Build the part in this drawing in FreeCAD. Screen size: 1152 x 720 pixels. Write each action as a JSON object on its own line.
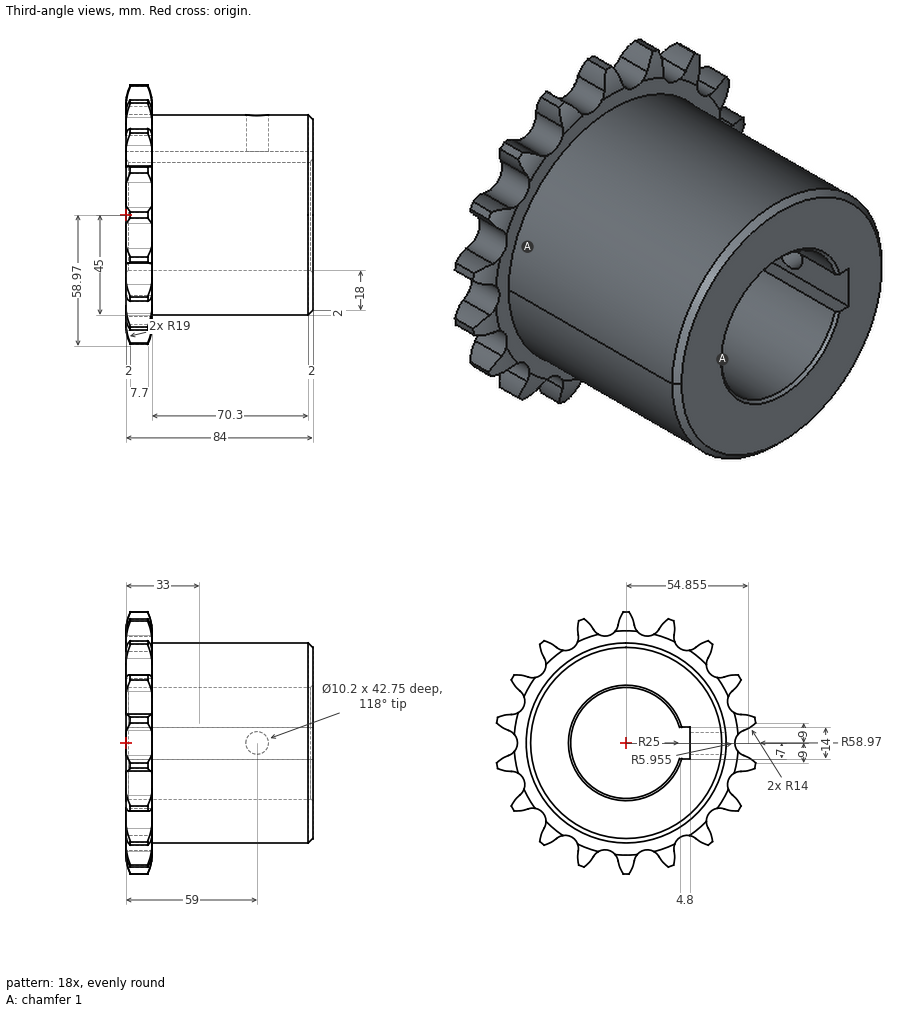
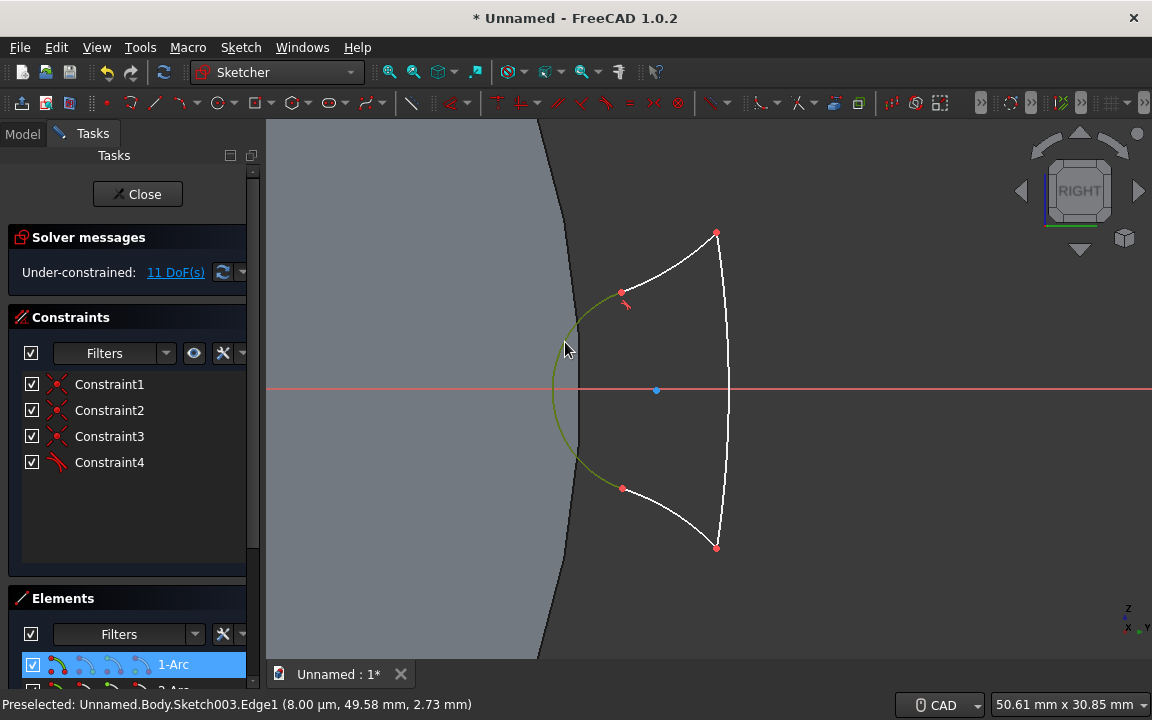
{"action": "left_click", "coordinate": [692, 526]}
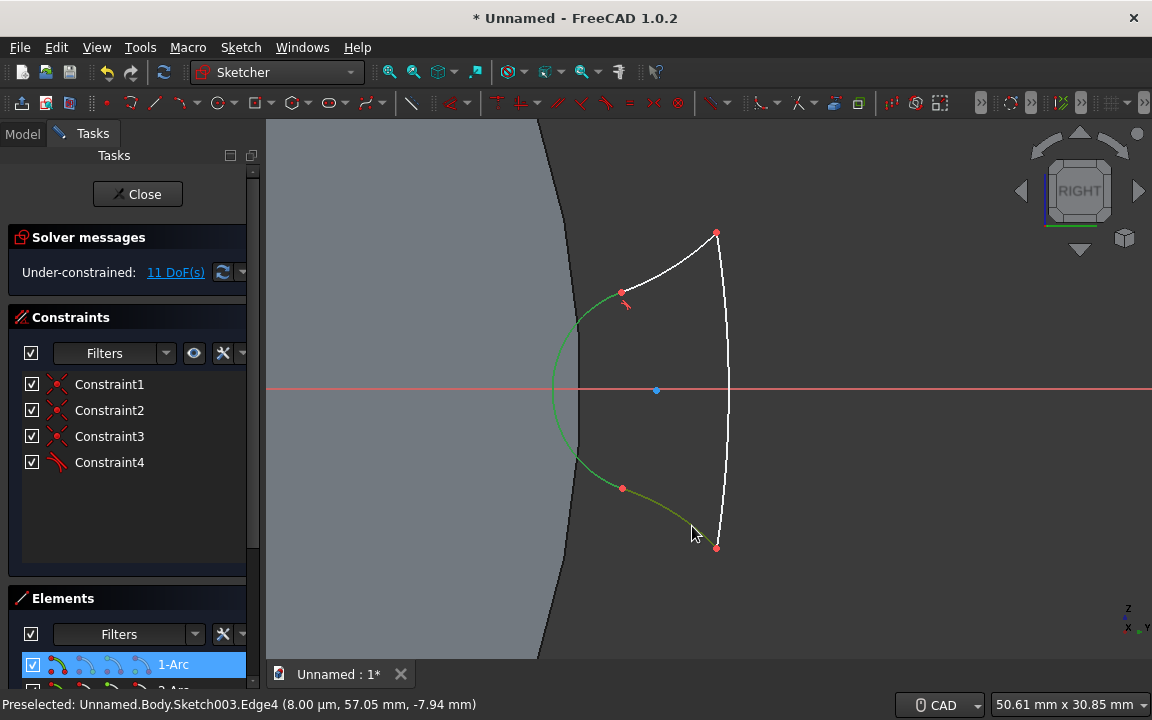
{"action": "left_click", "coordinate": [606, 104]}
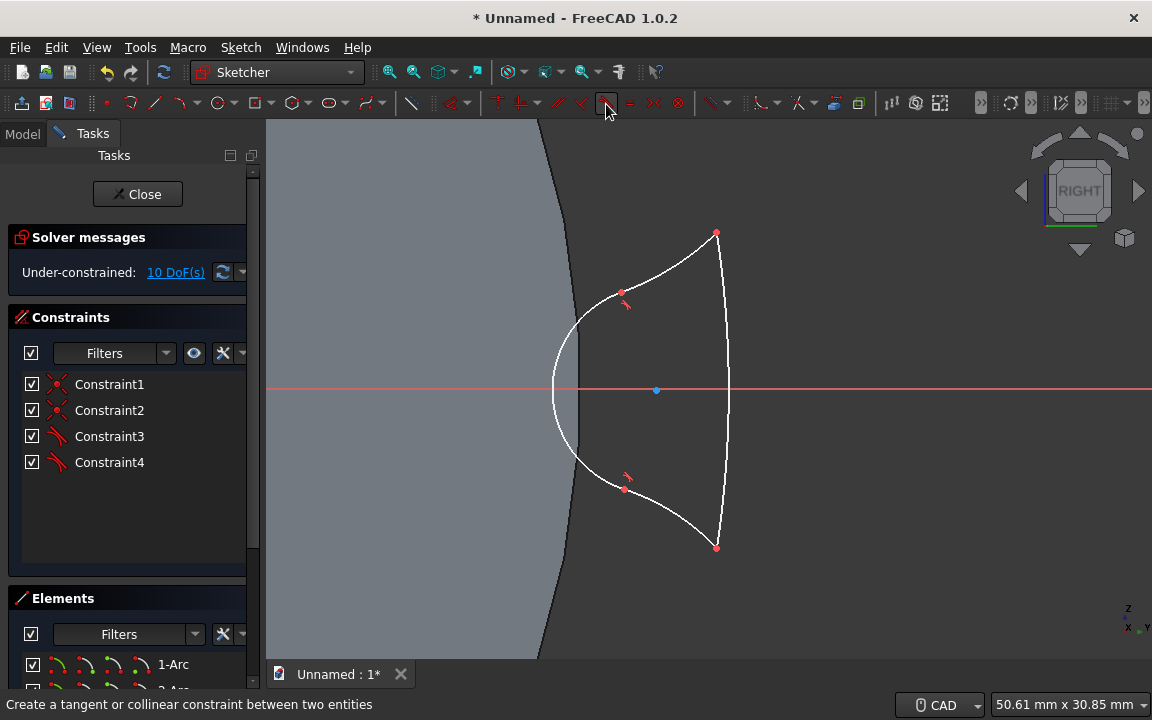
{"action": "scroll", "coordinate": [987, 389], "scroll_direction": "down", "scroll_amount": 4}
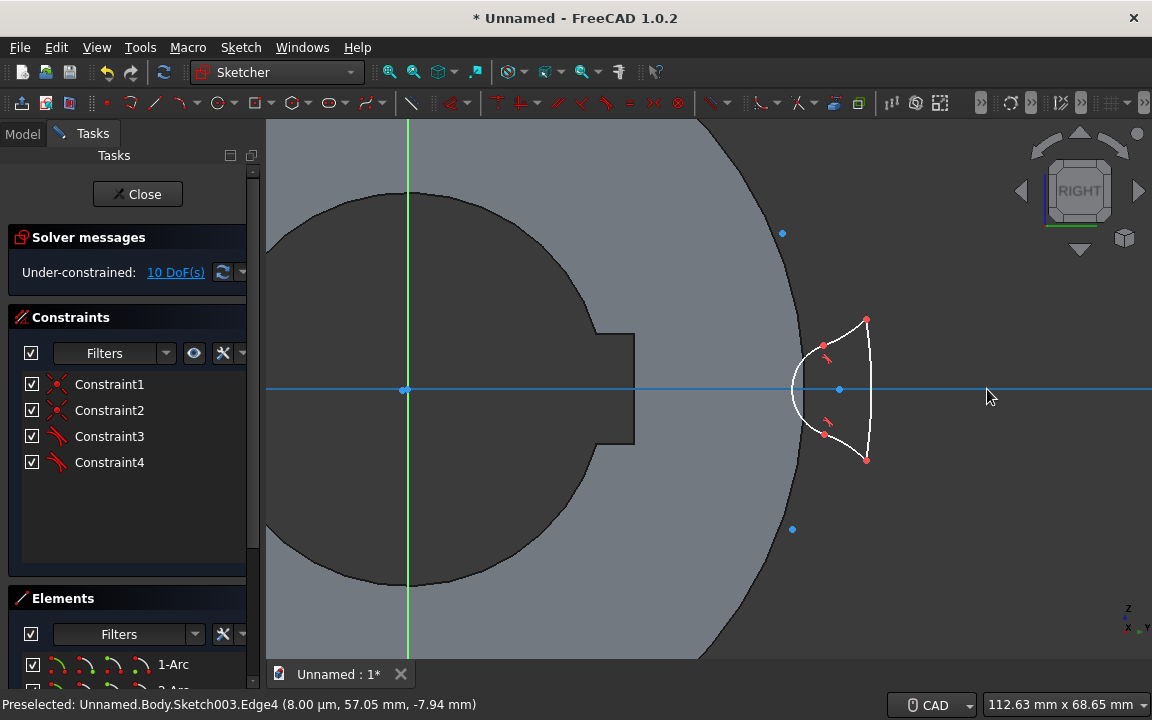
{"action": "left_click_drag", "start_coordinate": [393, 379], "coordinate": [418, 400]}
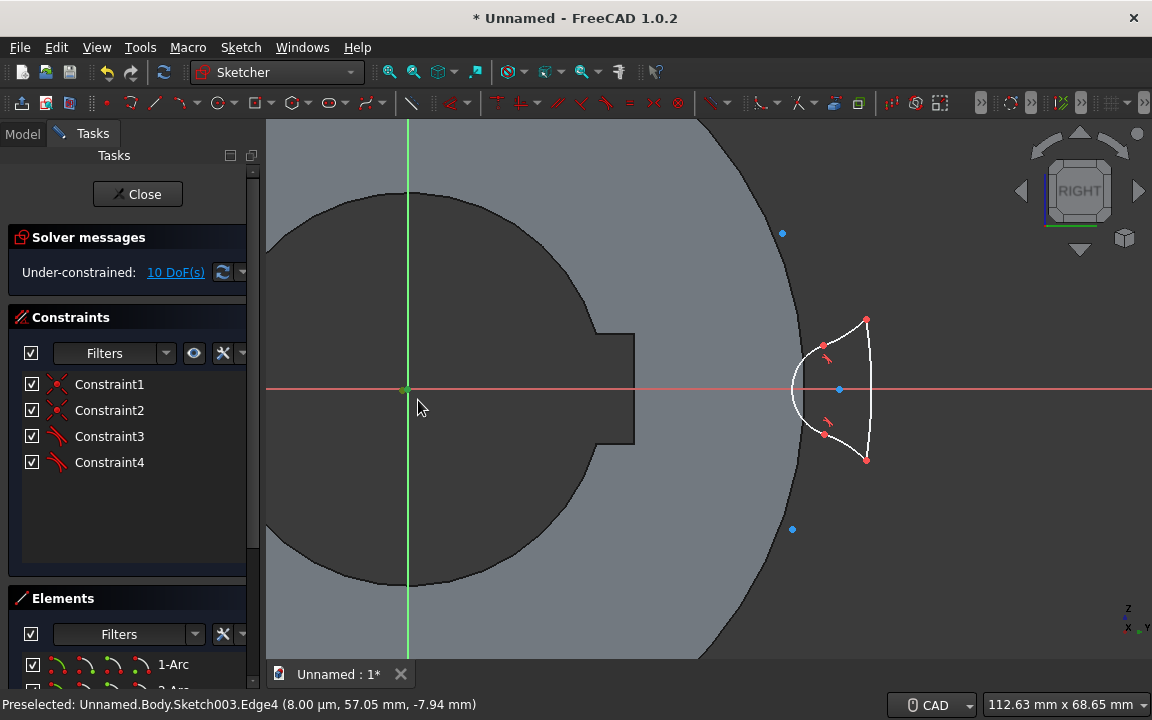
{"action": "key", "text": "c"}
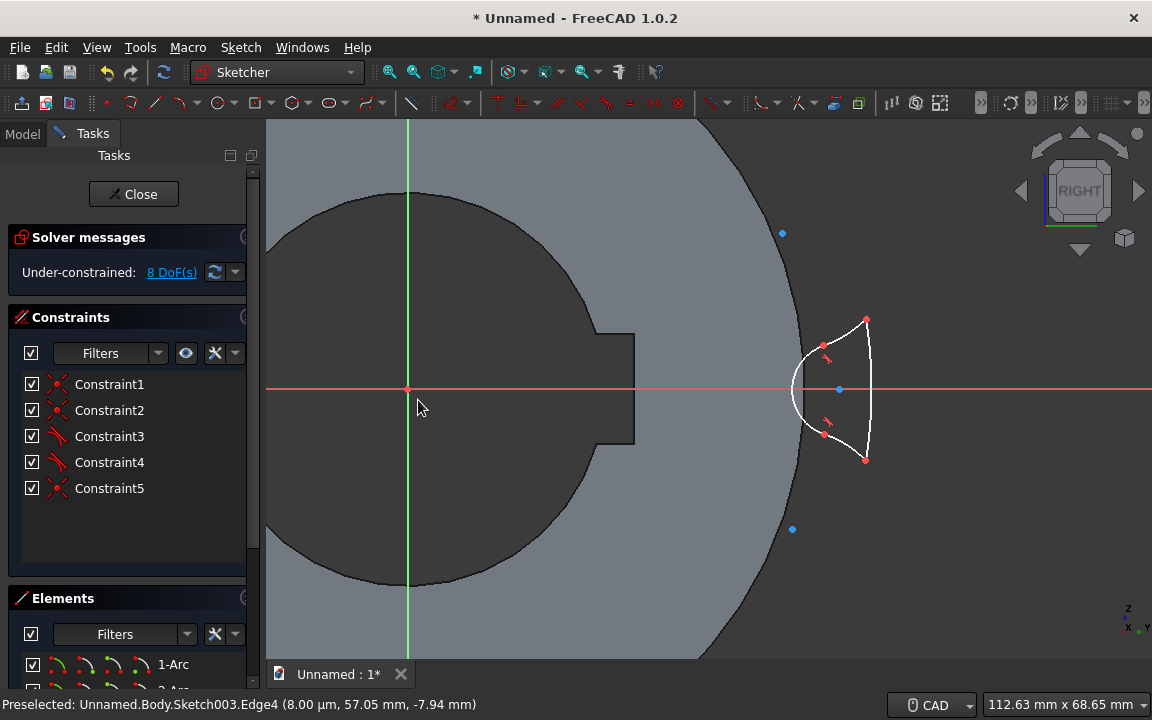
{"action": "left_click", "coordinate": [837, 340]}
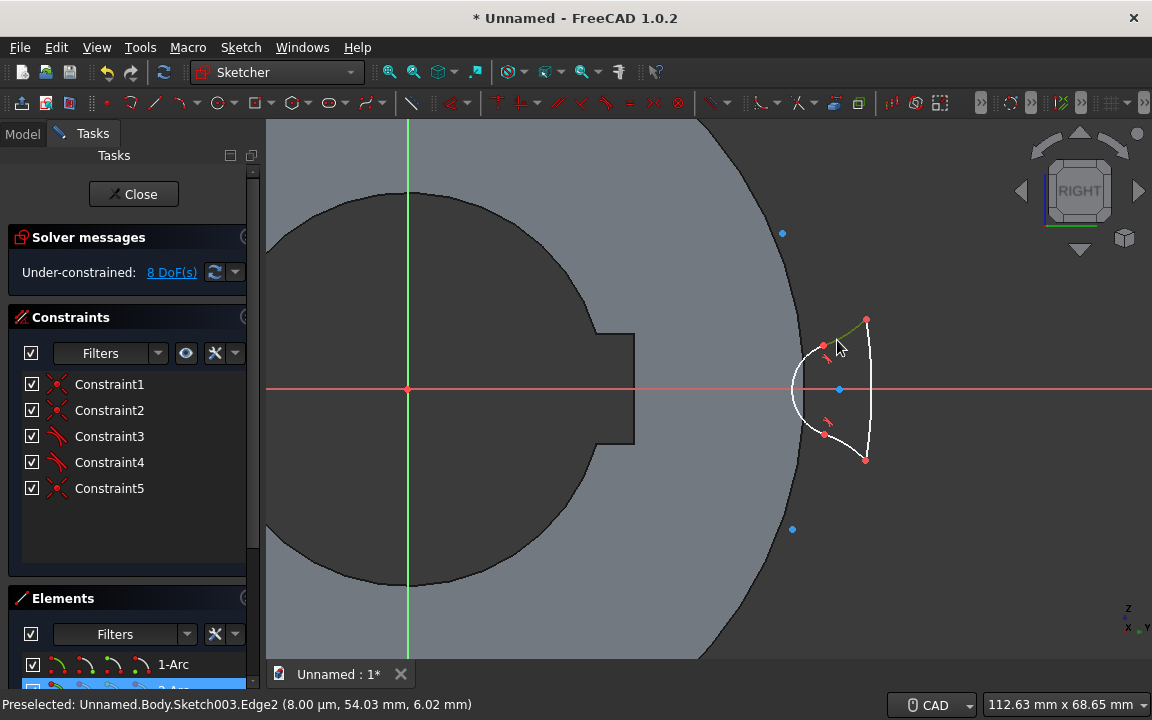
{"action": "left_click", "coordinate": [855, 451]}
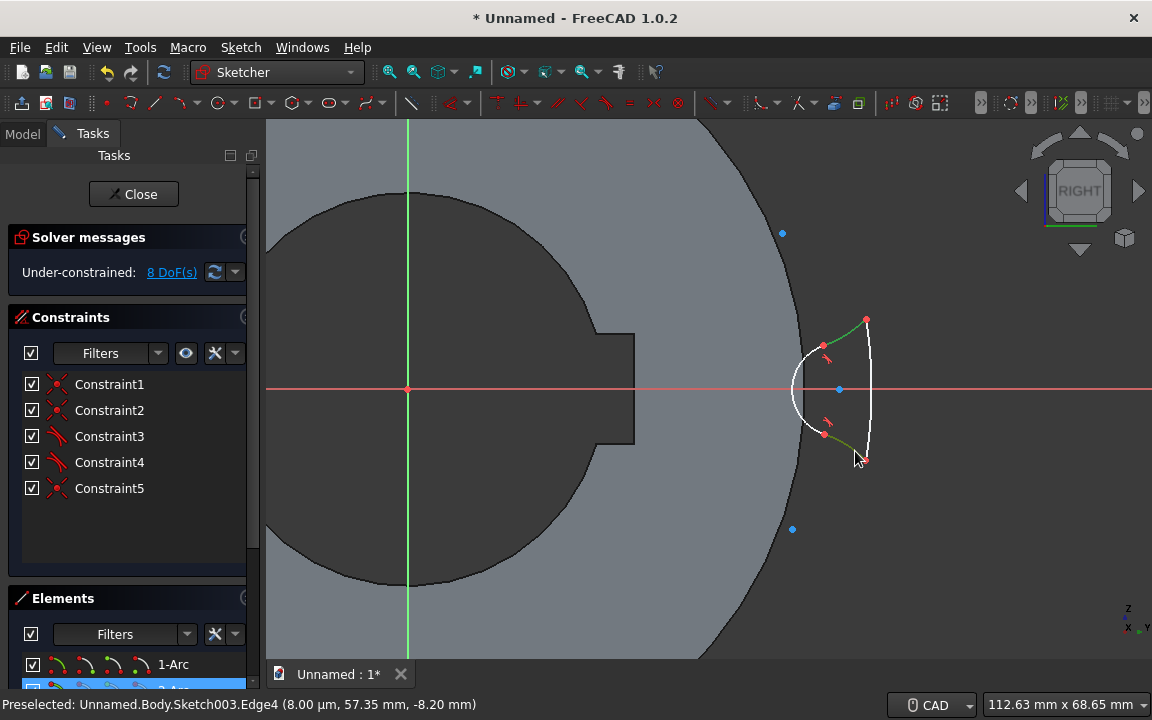
{"action": "key", "text": "e"}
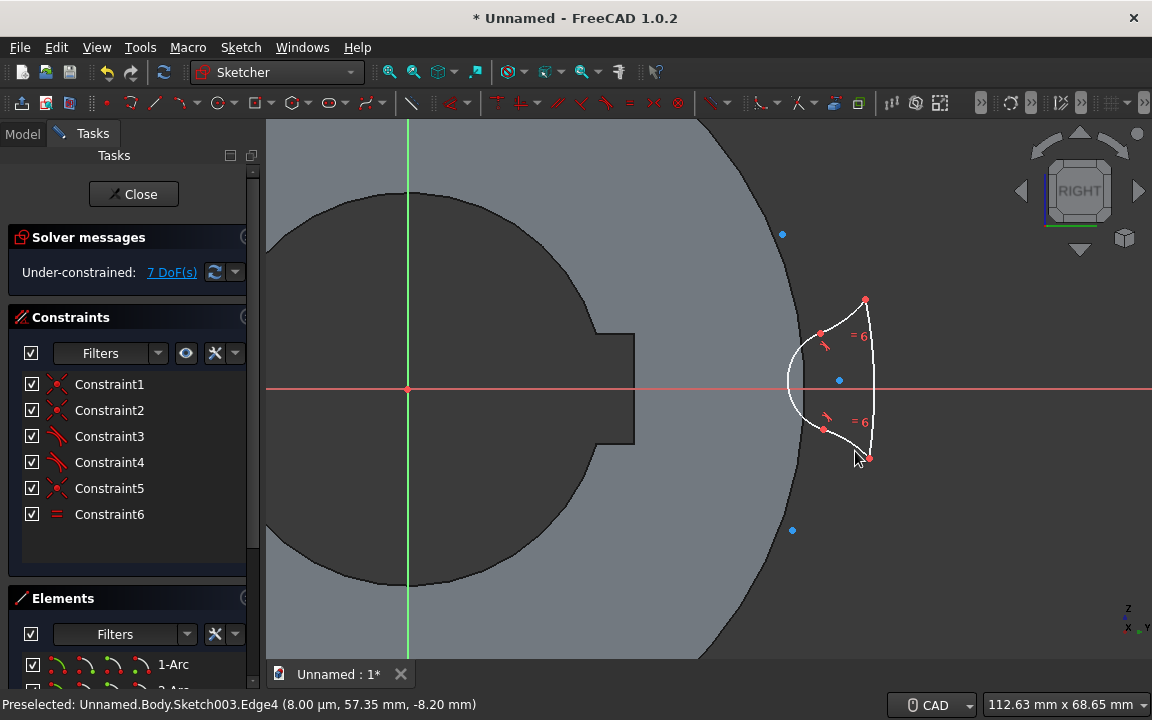
{"action": "left_click", "coordinate": [839, 381]}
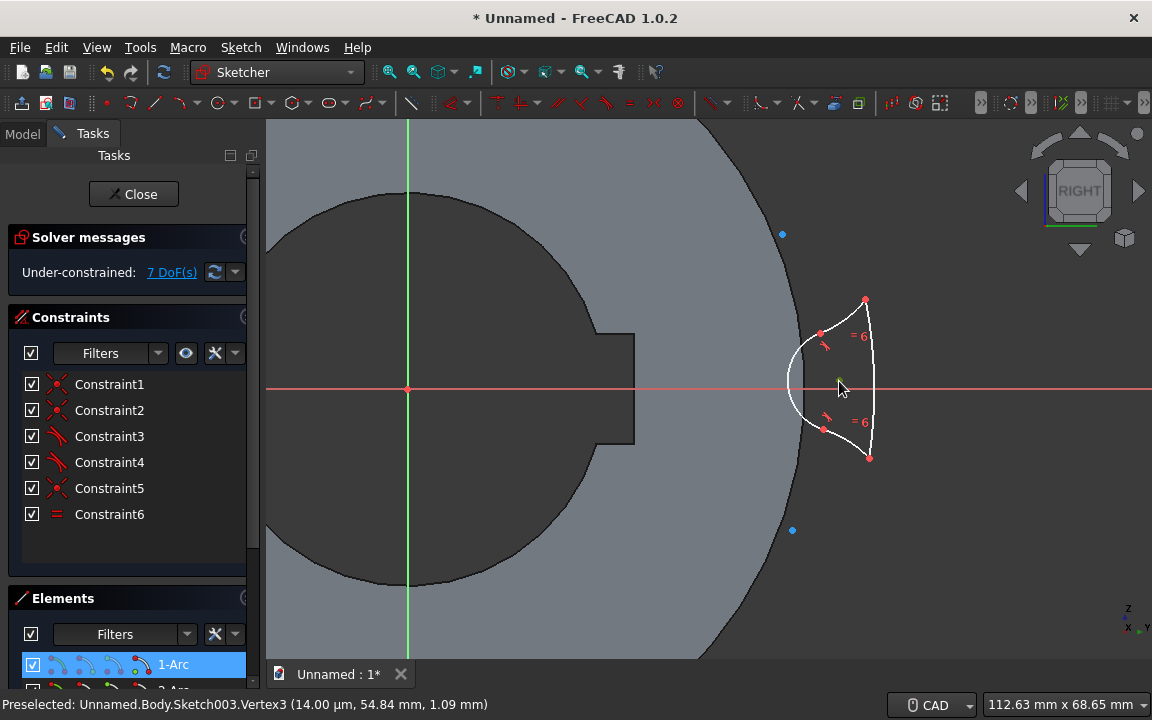
{"action": "left_click", "coordinate": [344, 389]}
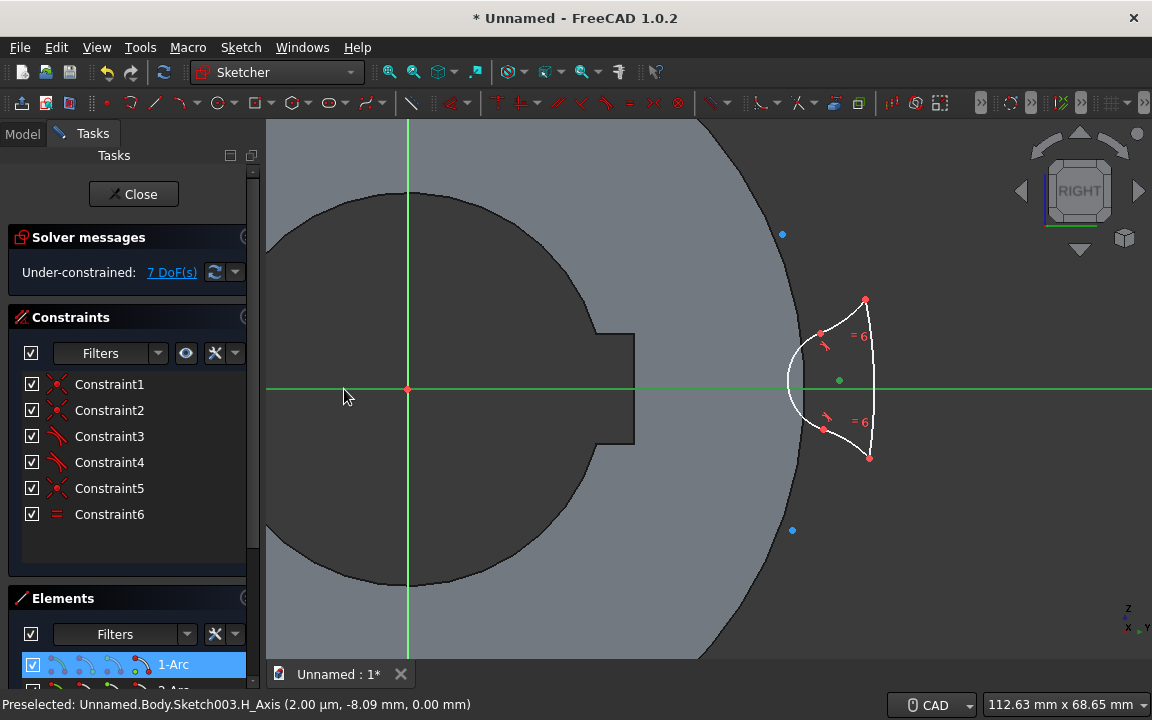
{"action": "key", "text": "c"}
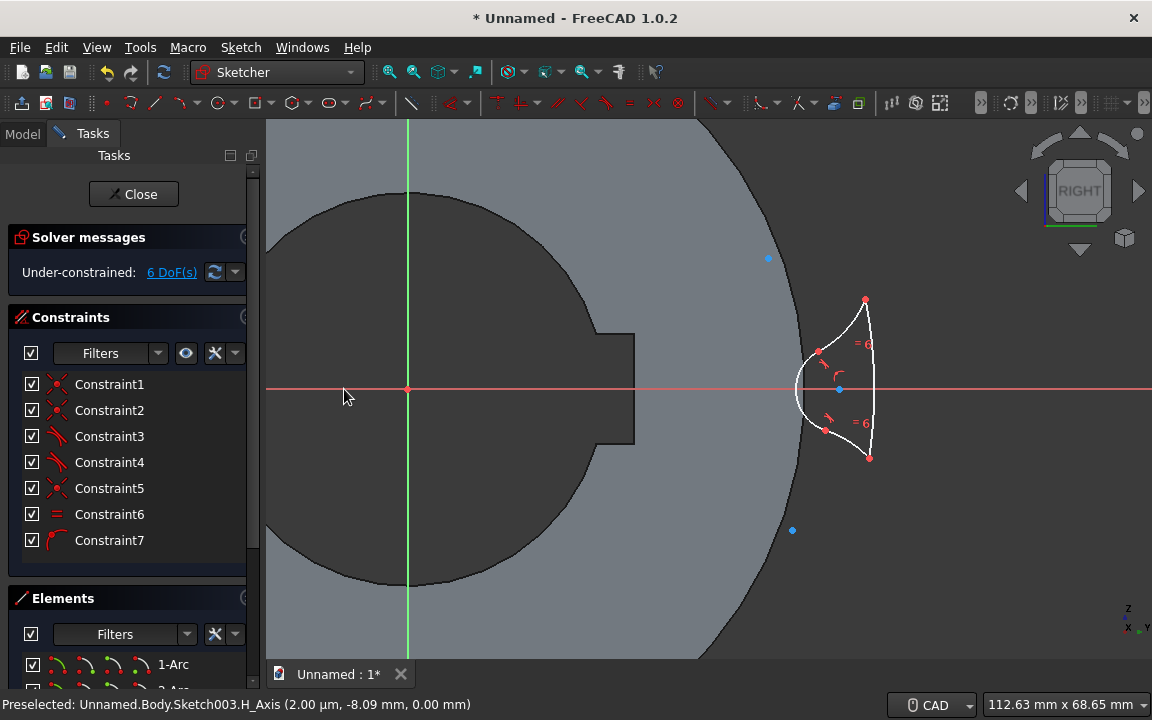
{"action": "left_click", "coordinate": [450, 104]}